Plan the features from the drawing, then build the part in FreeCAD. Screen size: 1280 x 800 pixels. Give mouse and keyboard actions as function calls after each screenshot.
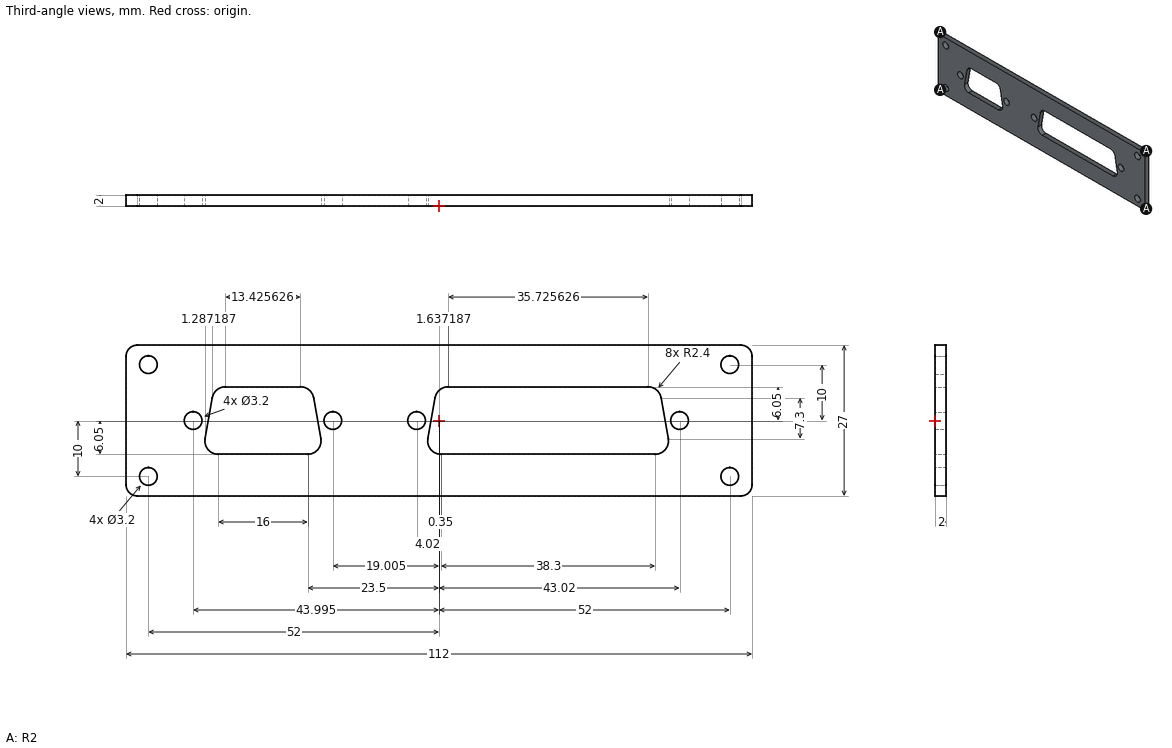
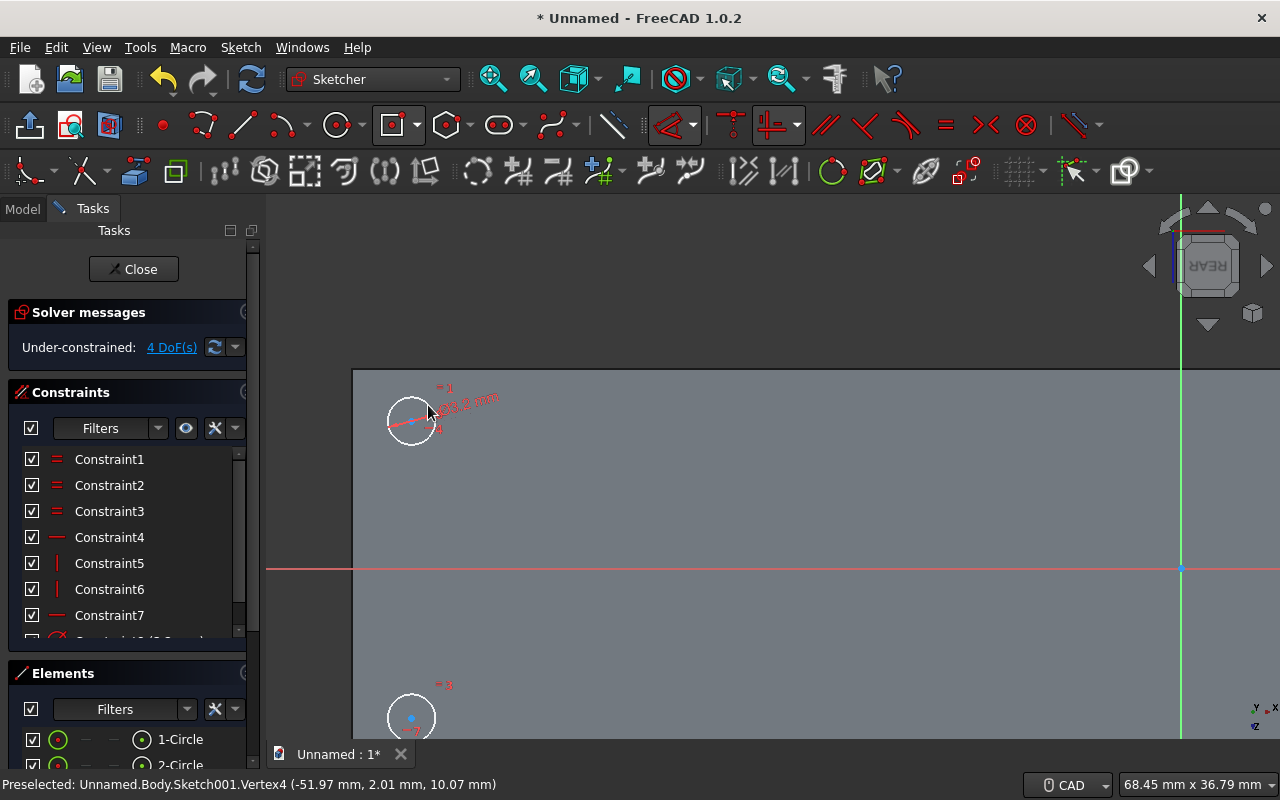
click(412, 421)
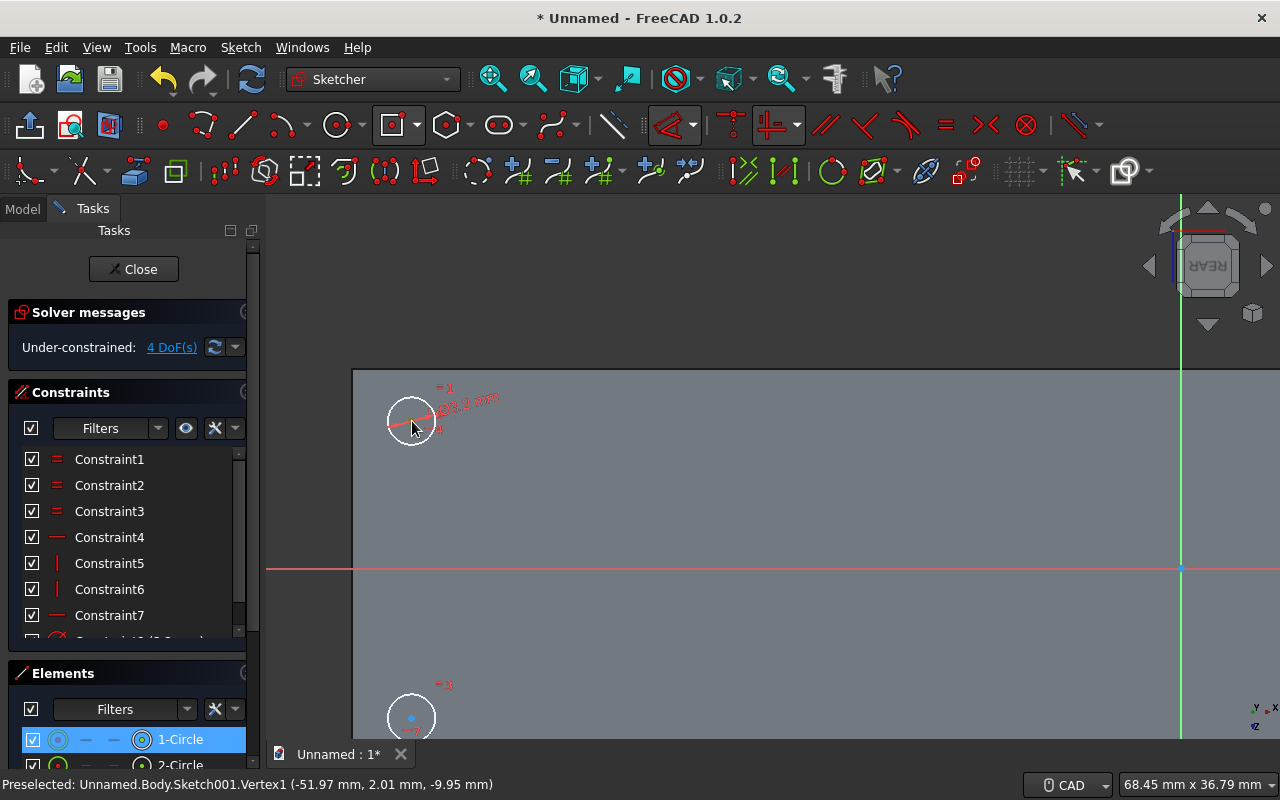
click(696, 126)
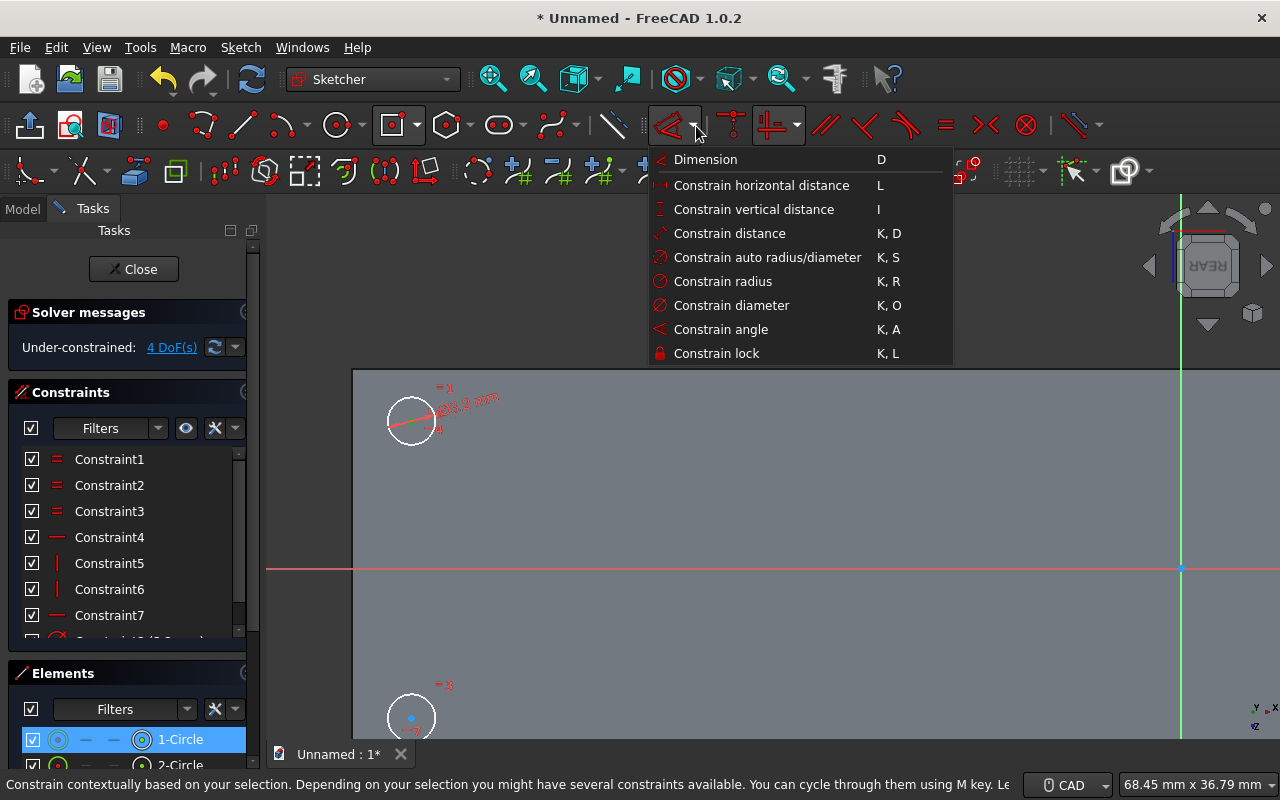
click(801, 185)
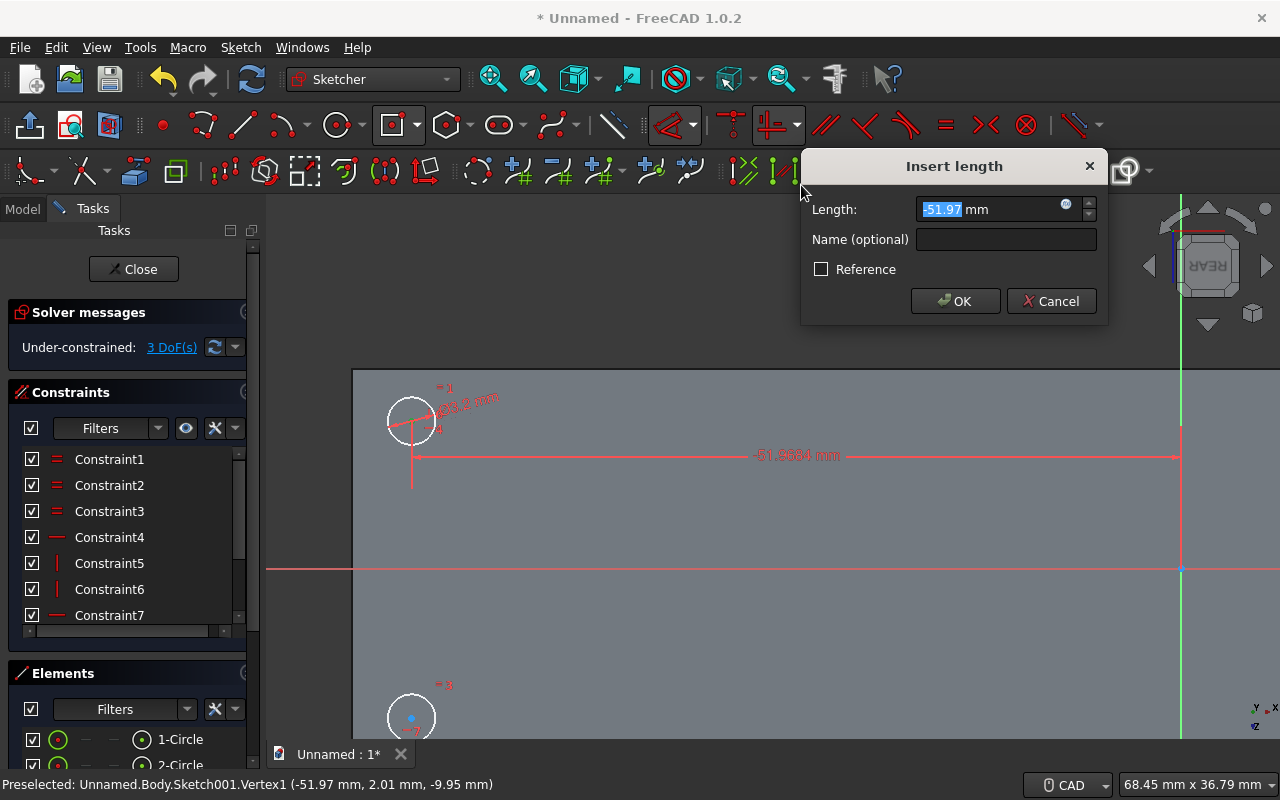
text(-52)
key(Return)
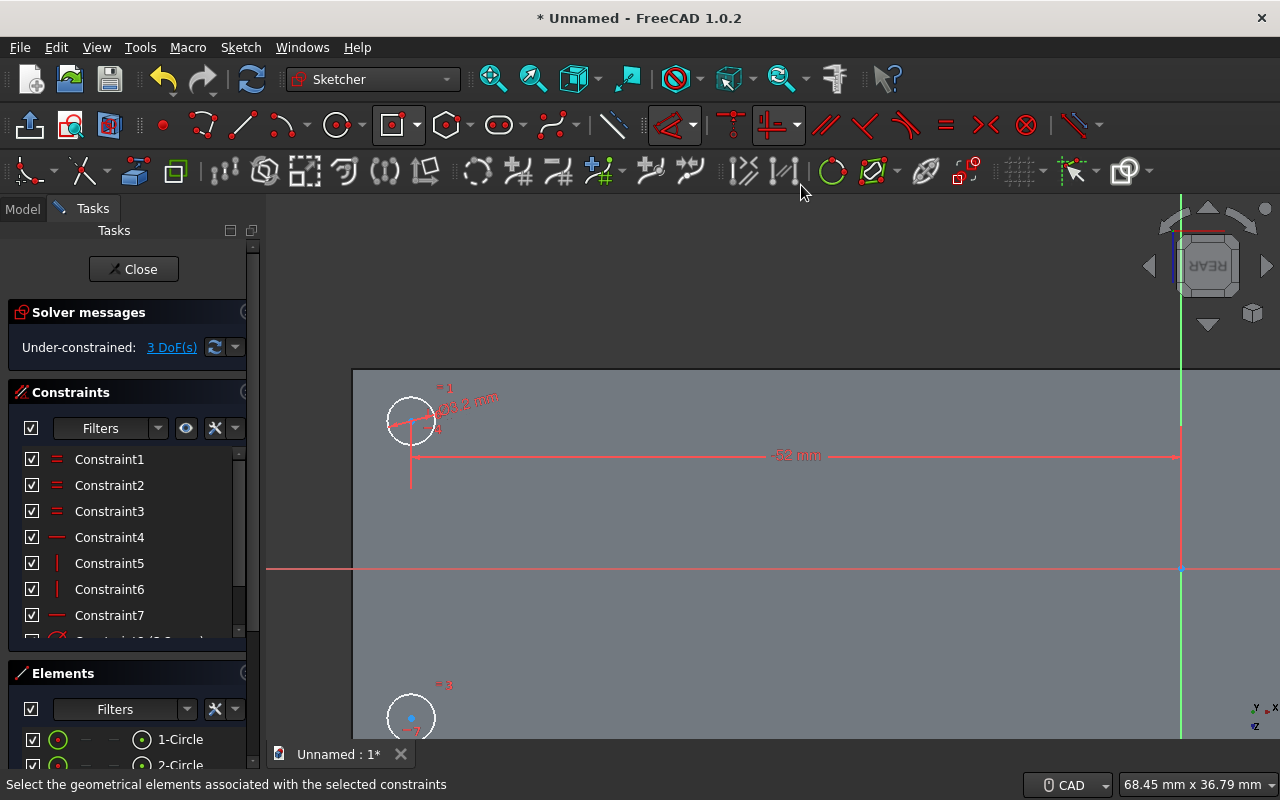
click(411, 421)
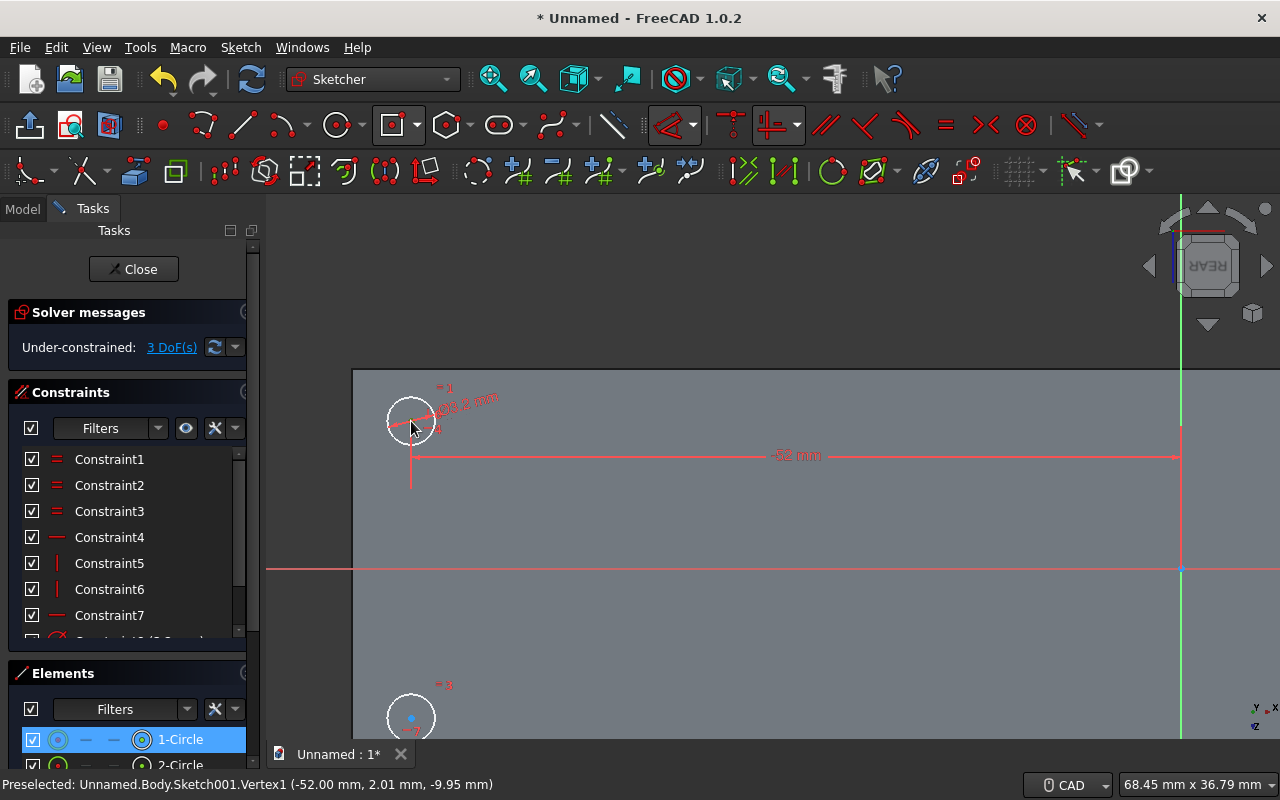
click(696, 126)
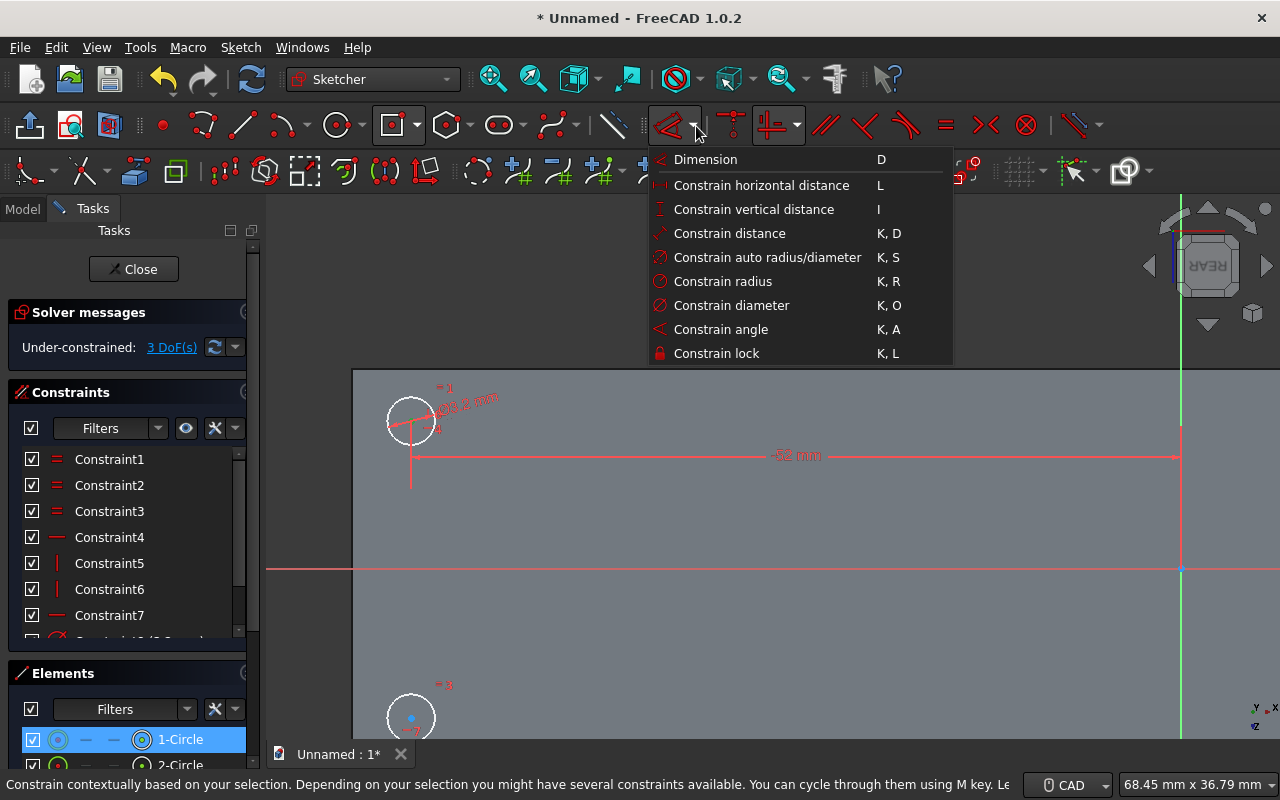
click(801, 209)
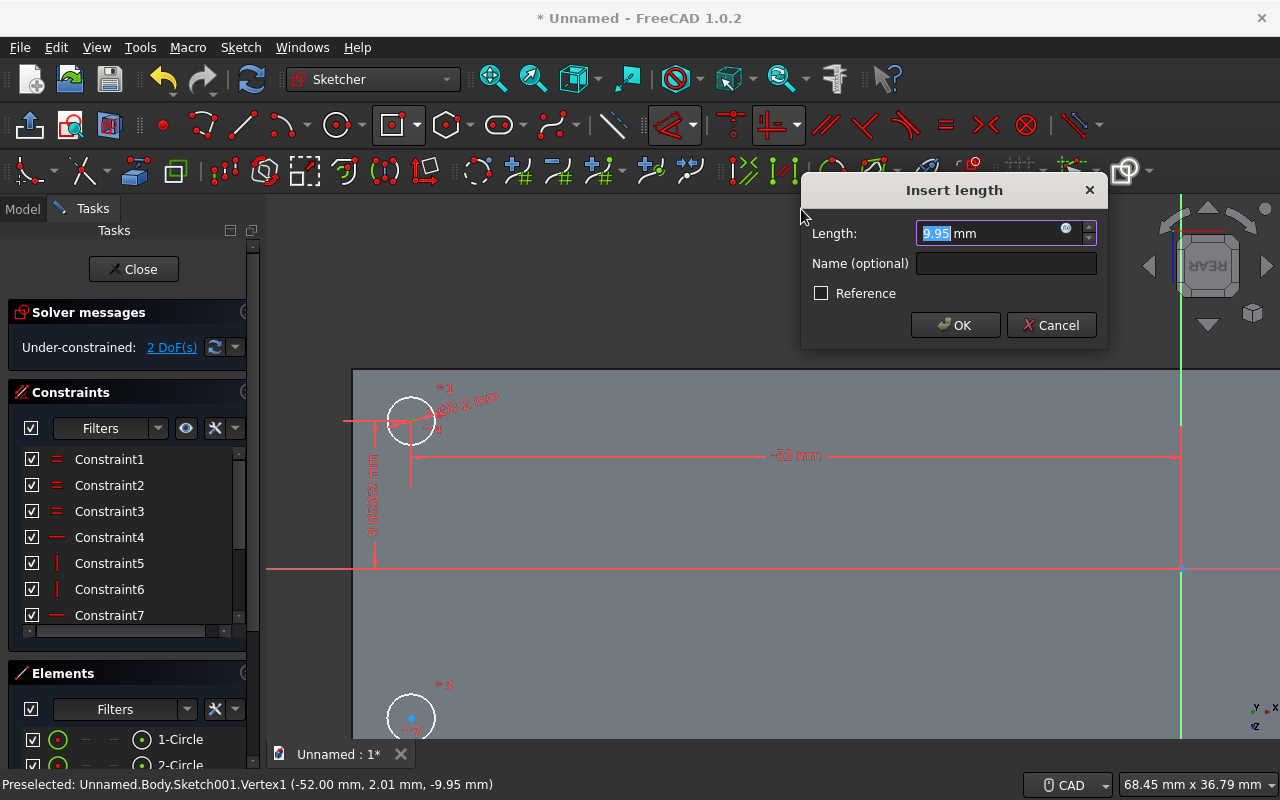
text(10)
key(Return)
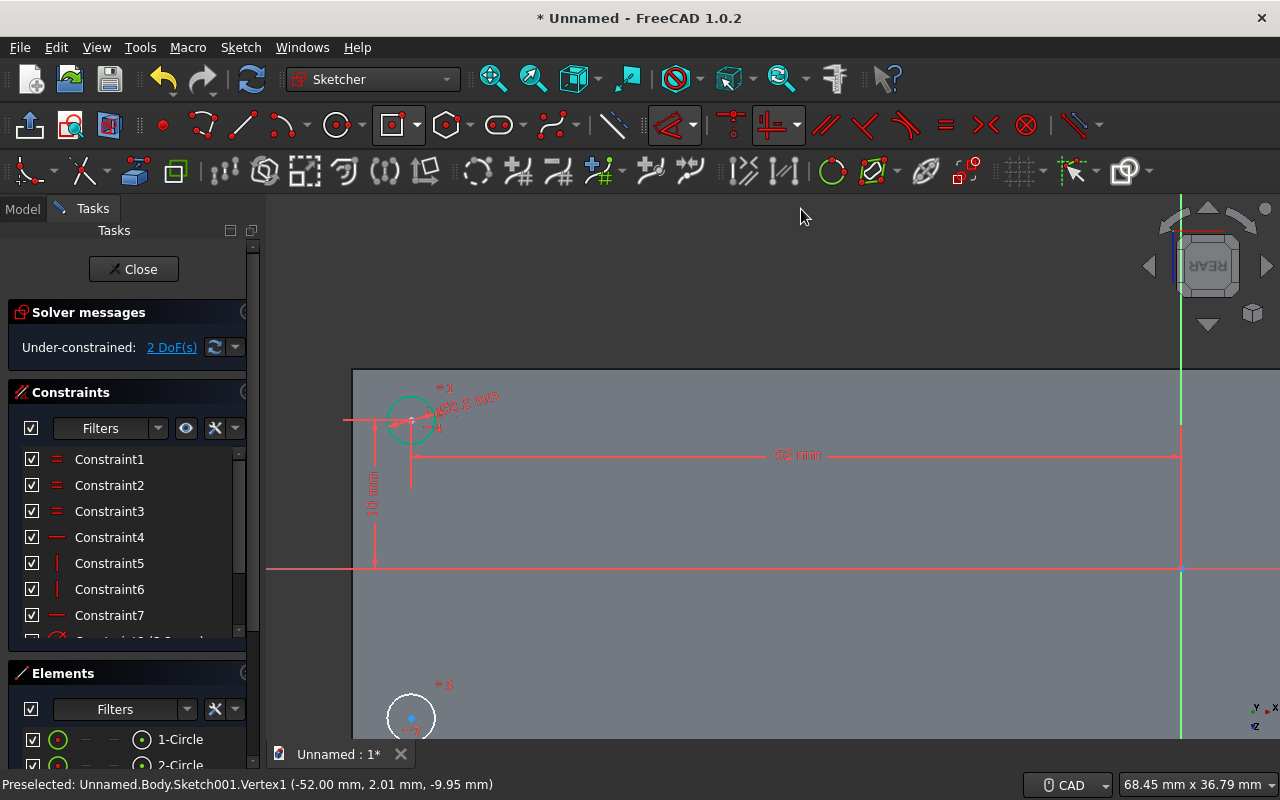
scroll(427, 407, down, 5)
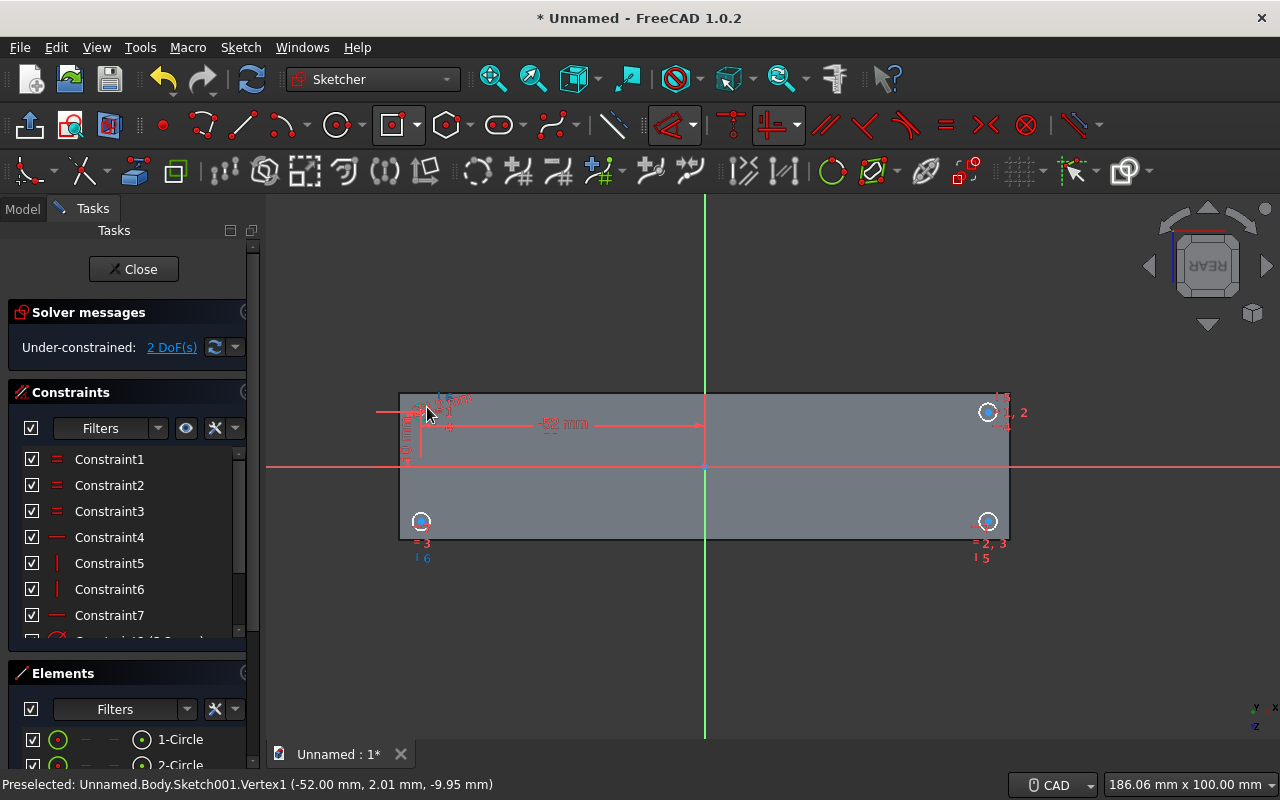
click(988, 412)